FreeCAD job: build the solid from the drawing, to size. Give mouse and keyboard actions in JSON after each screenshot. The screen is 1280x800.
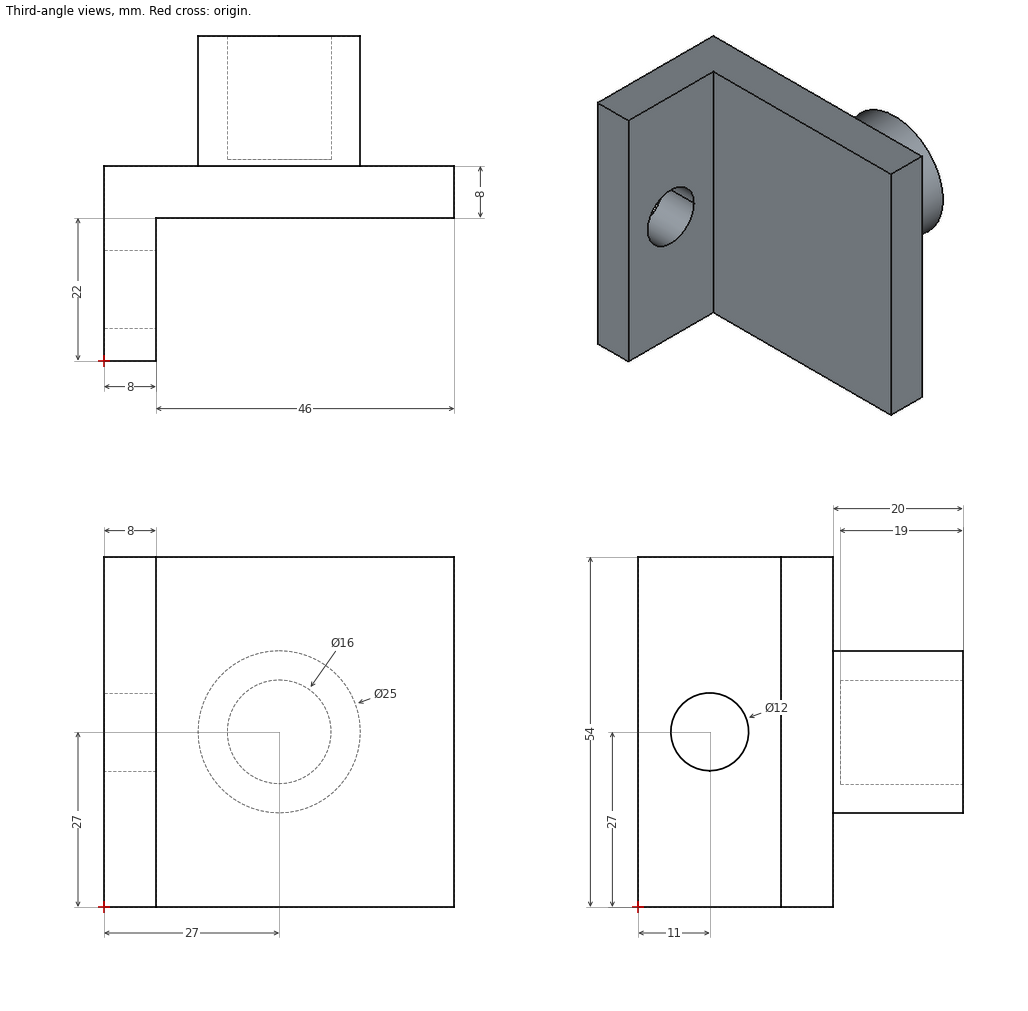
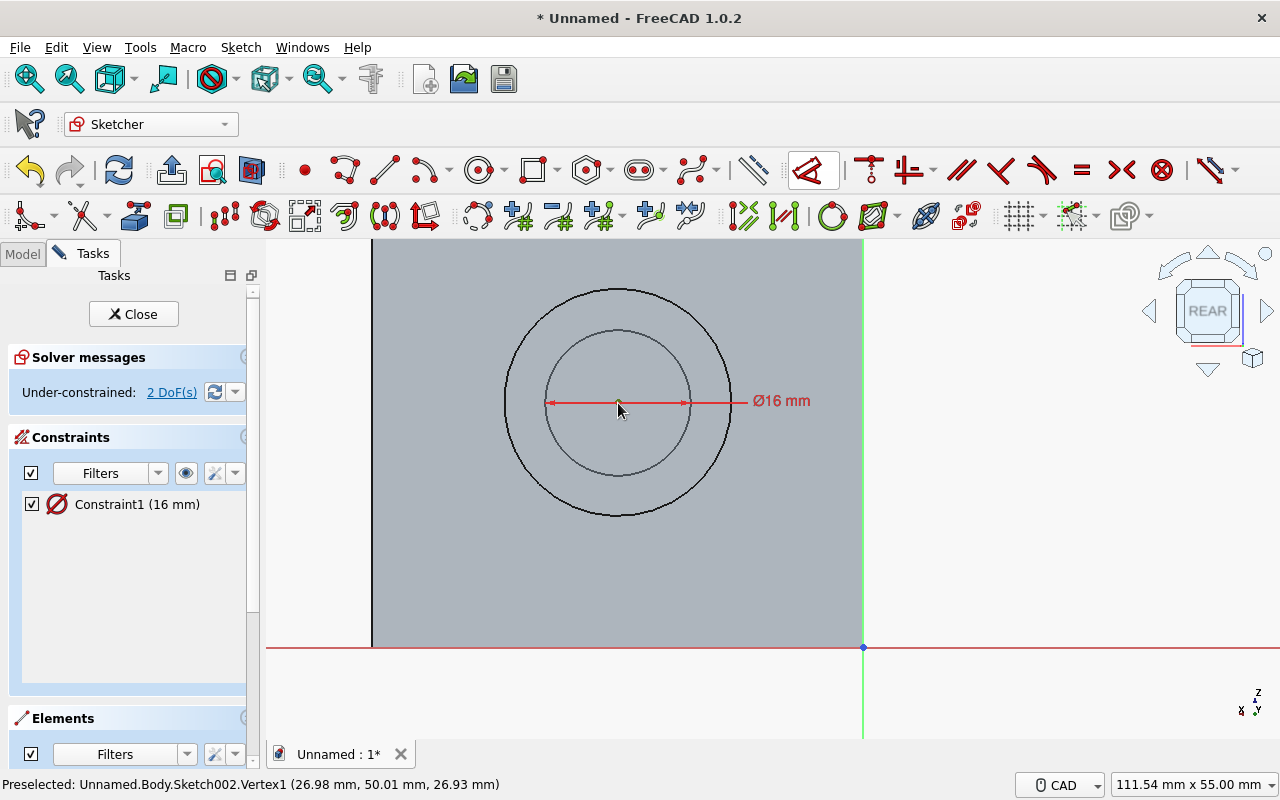
{"action": "key", "text": "l"}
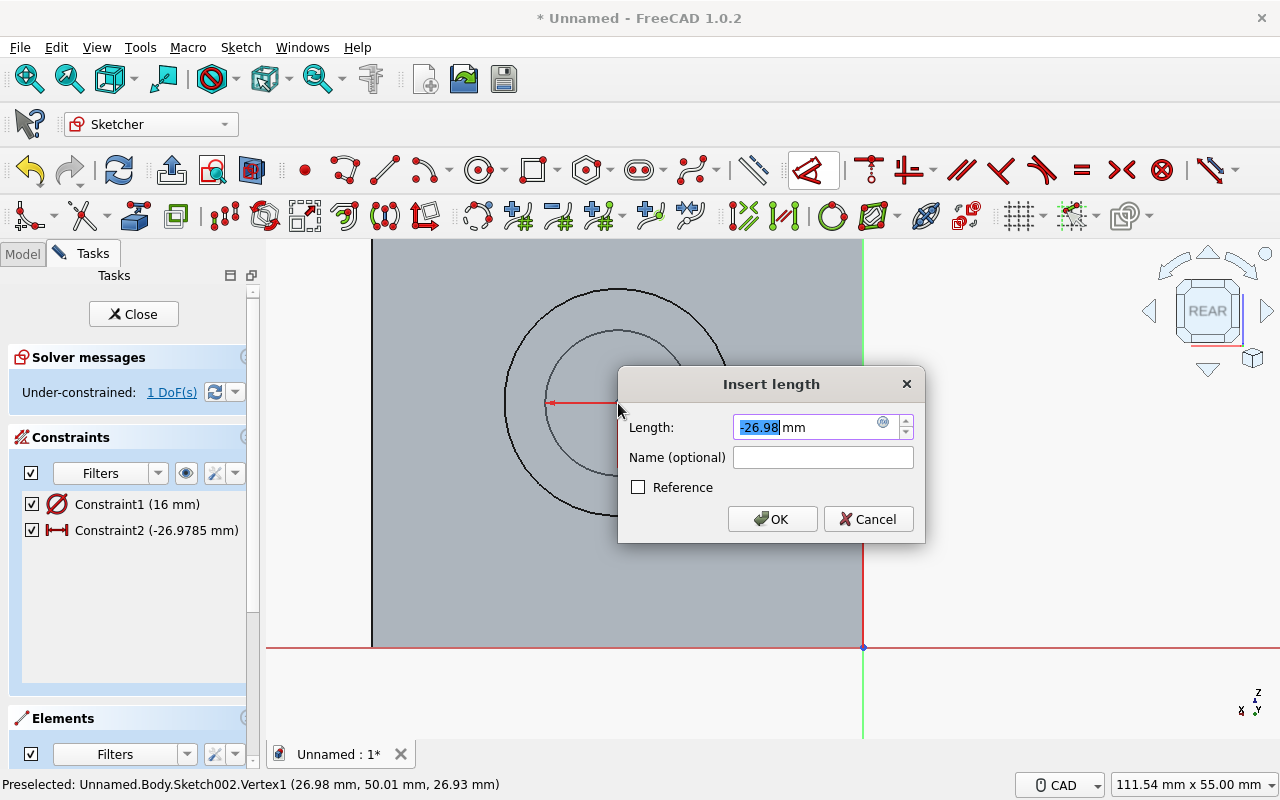
{"action": "type", "text": "-27"}
{"action": "key", "text": "Return"}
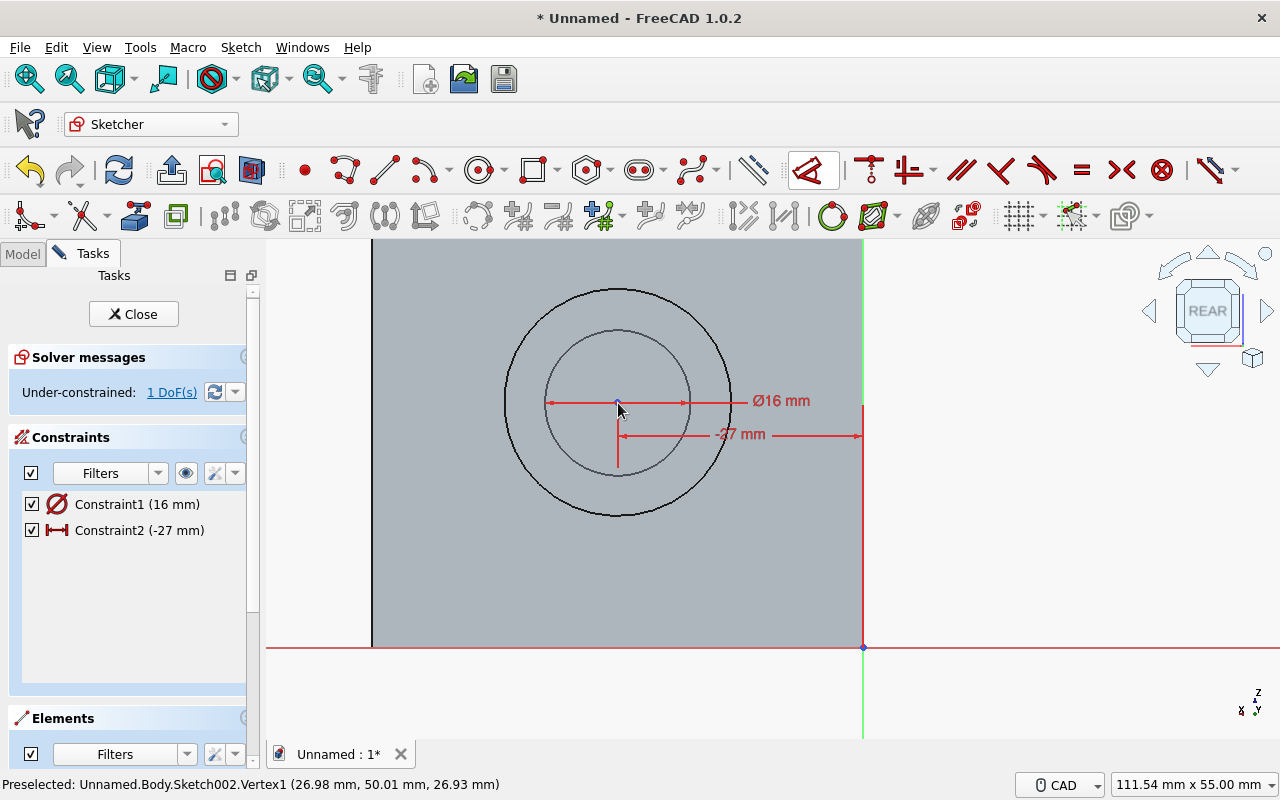
{"action": "left_click", "coordinate": [618, 403]}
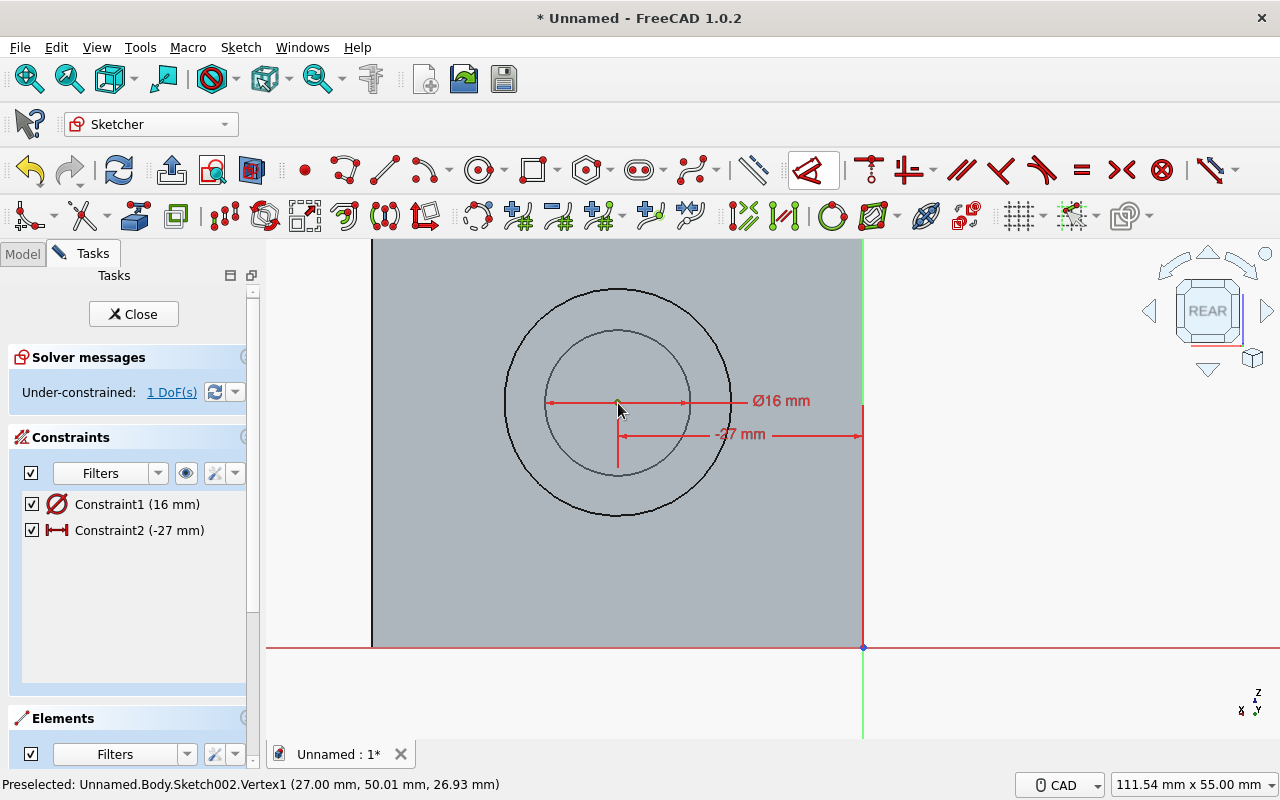
{"action": "key", "text": "i"}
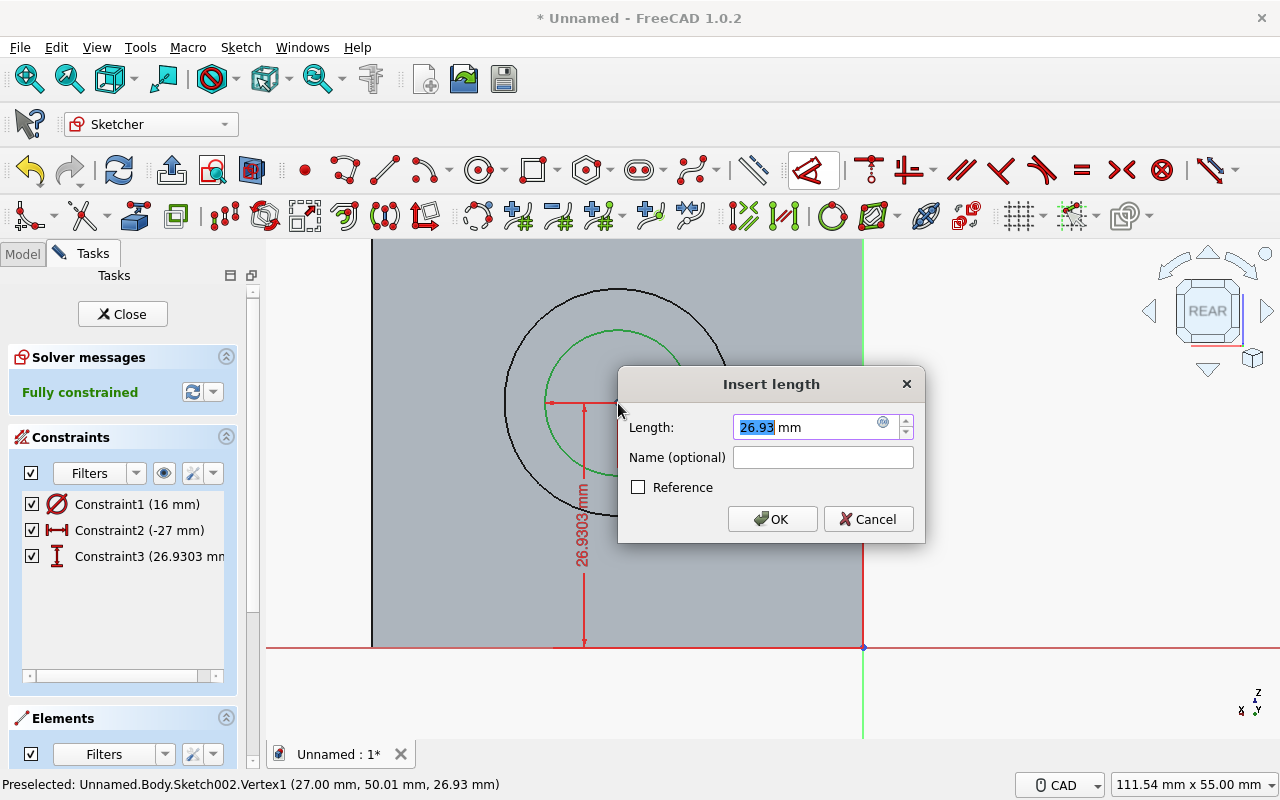
{"action": "type", "text": "27"}
{"action": "key", "text": "Return"}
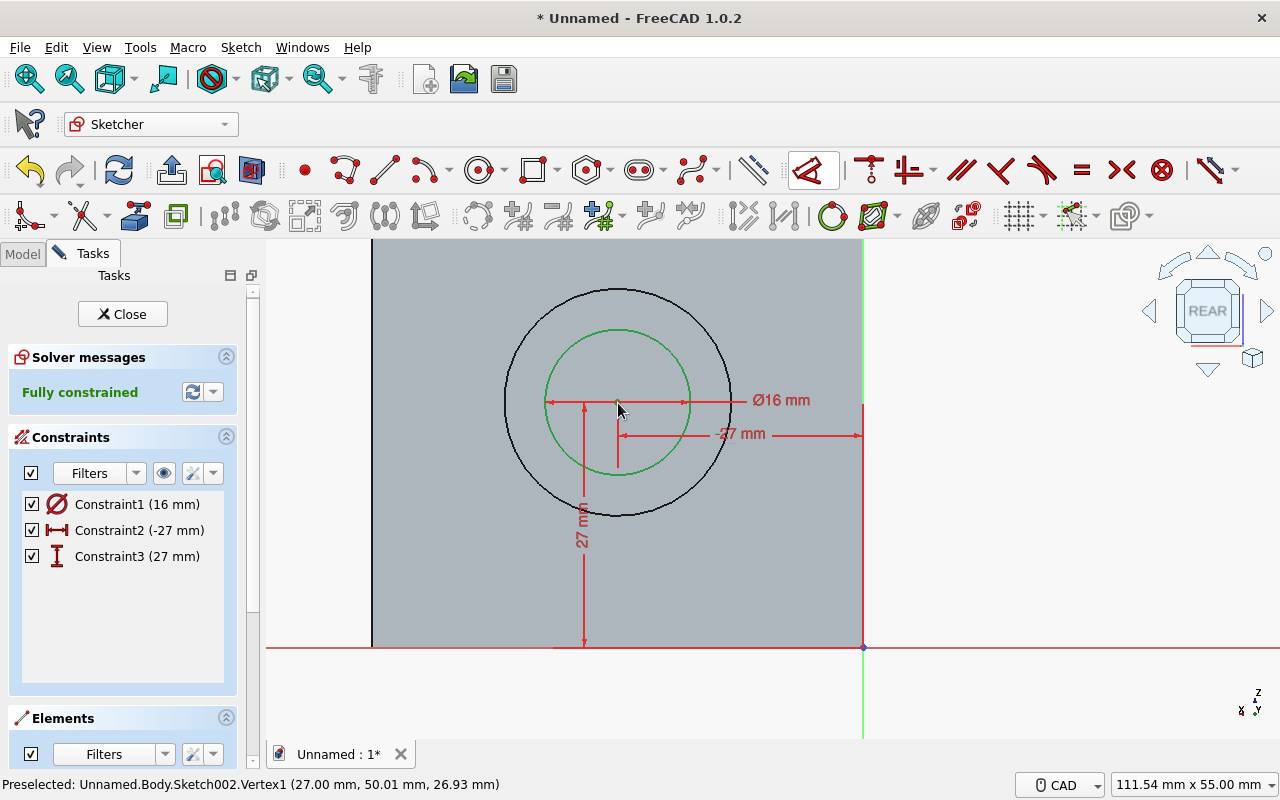
{"action": "left_click", "coordinate": [123, 314]}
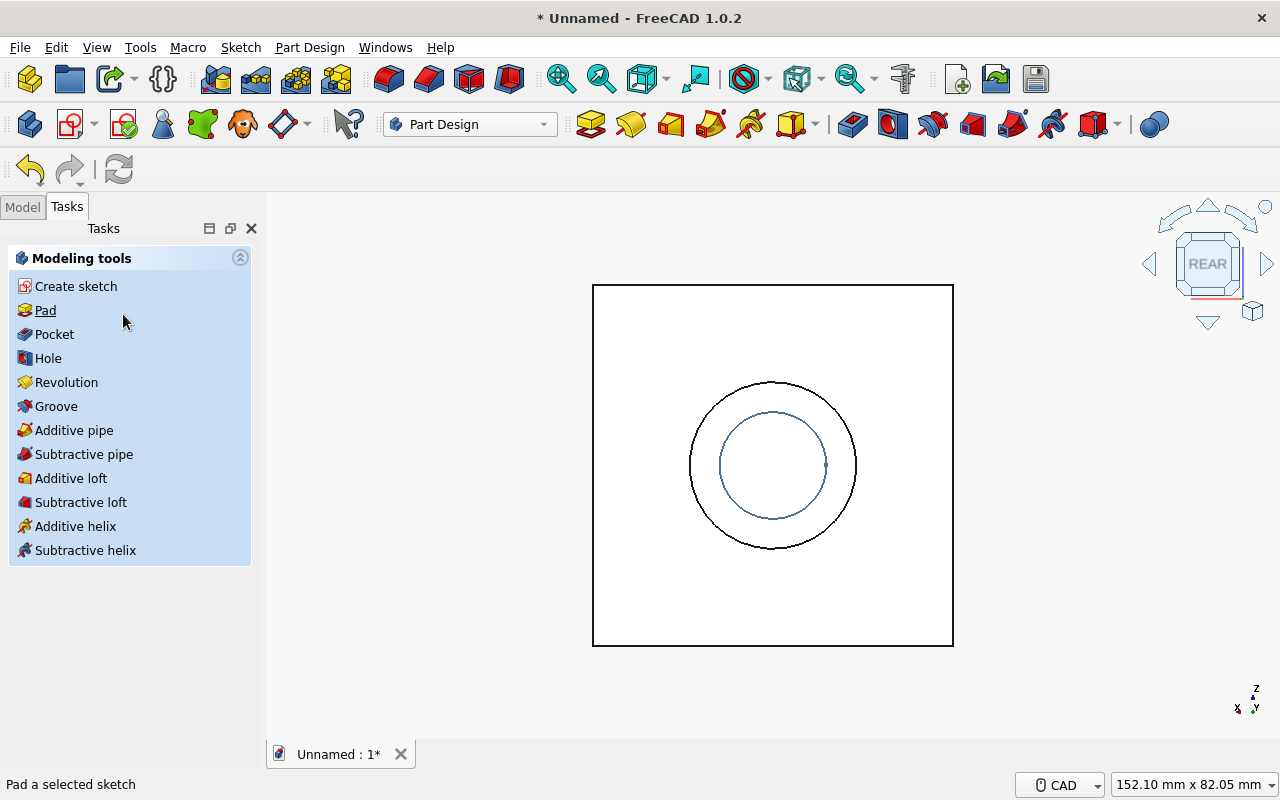
{"action": "left_click", "coordinate": [854, 124]}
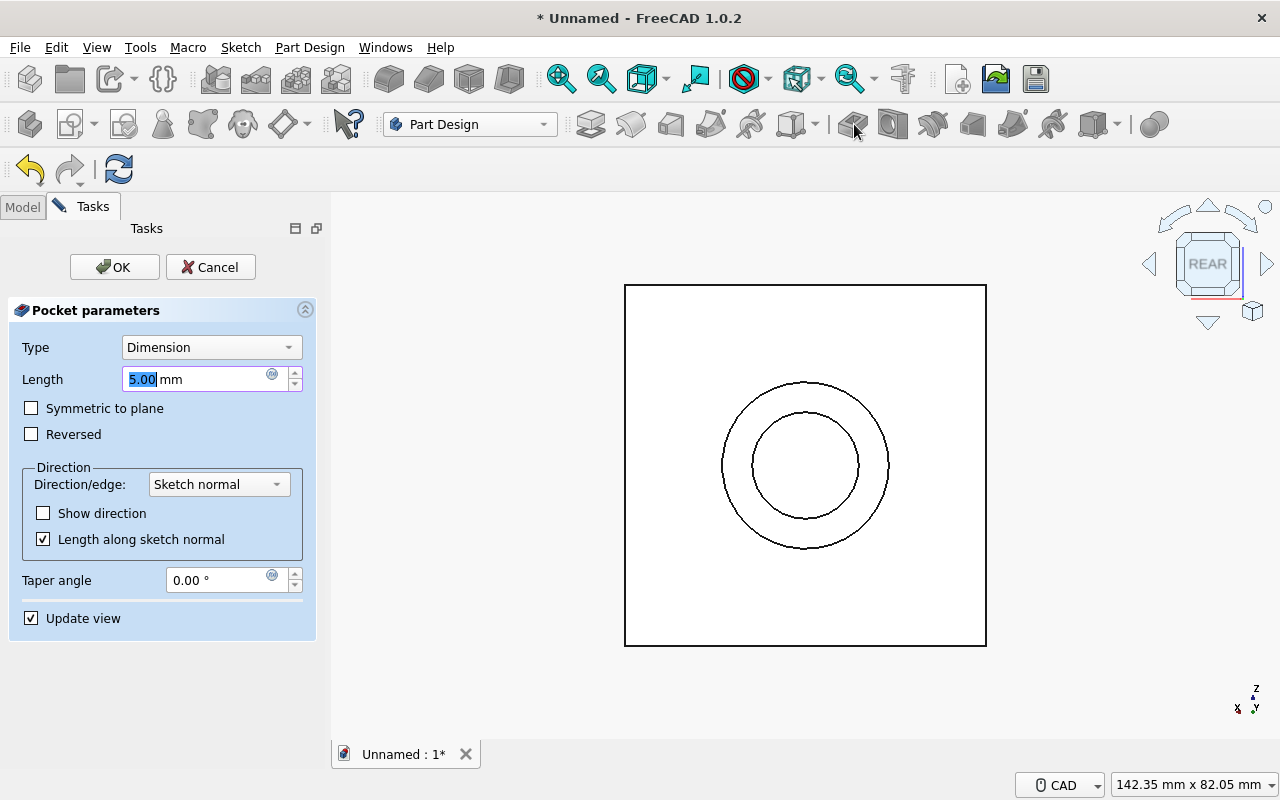
{"action": "type", "text": "19"}
{"action": "key", "text": "Tab"}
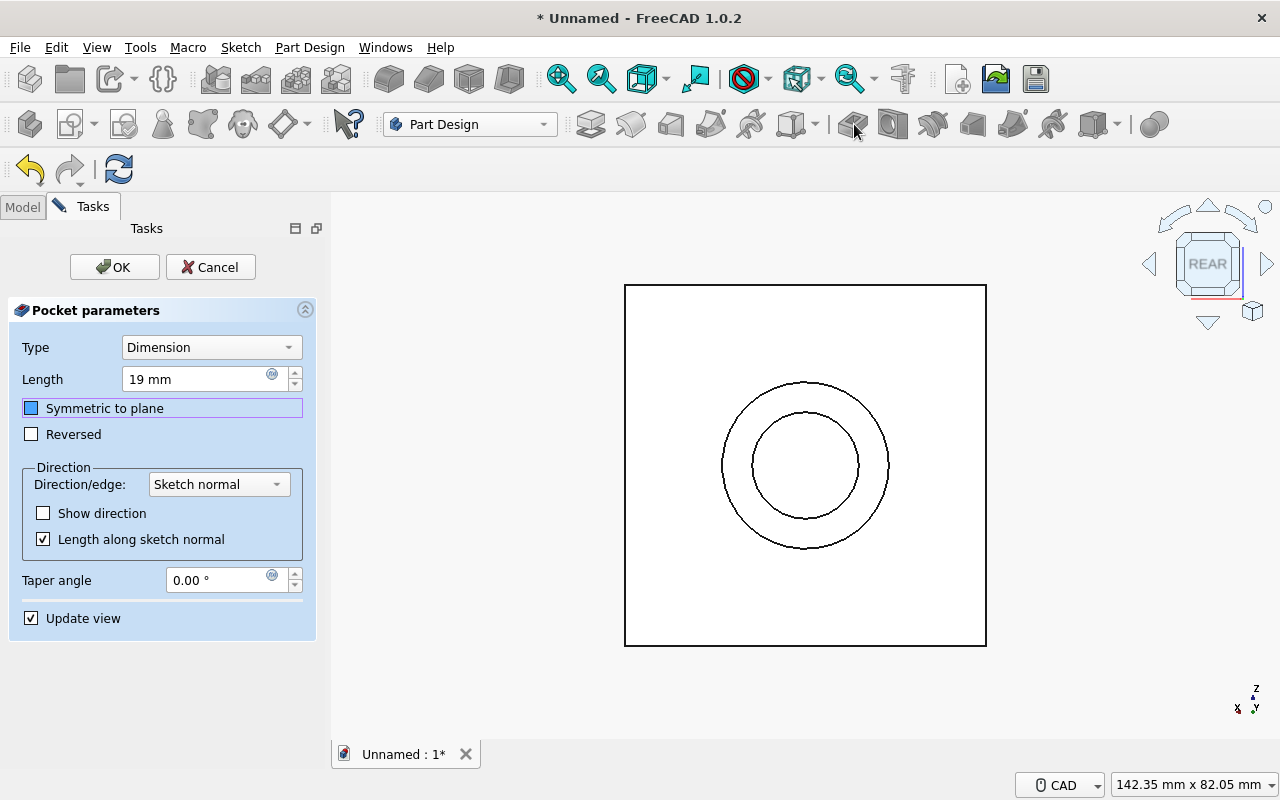
{"action": "left_click", "coordinate": [115, 267]}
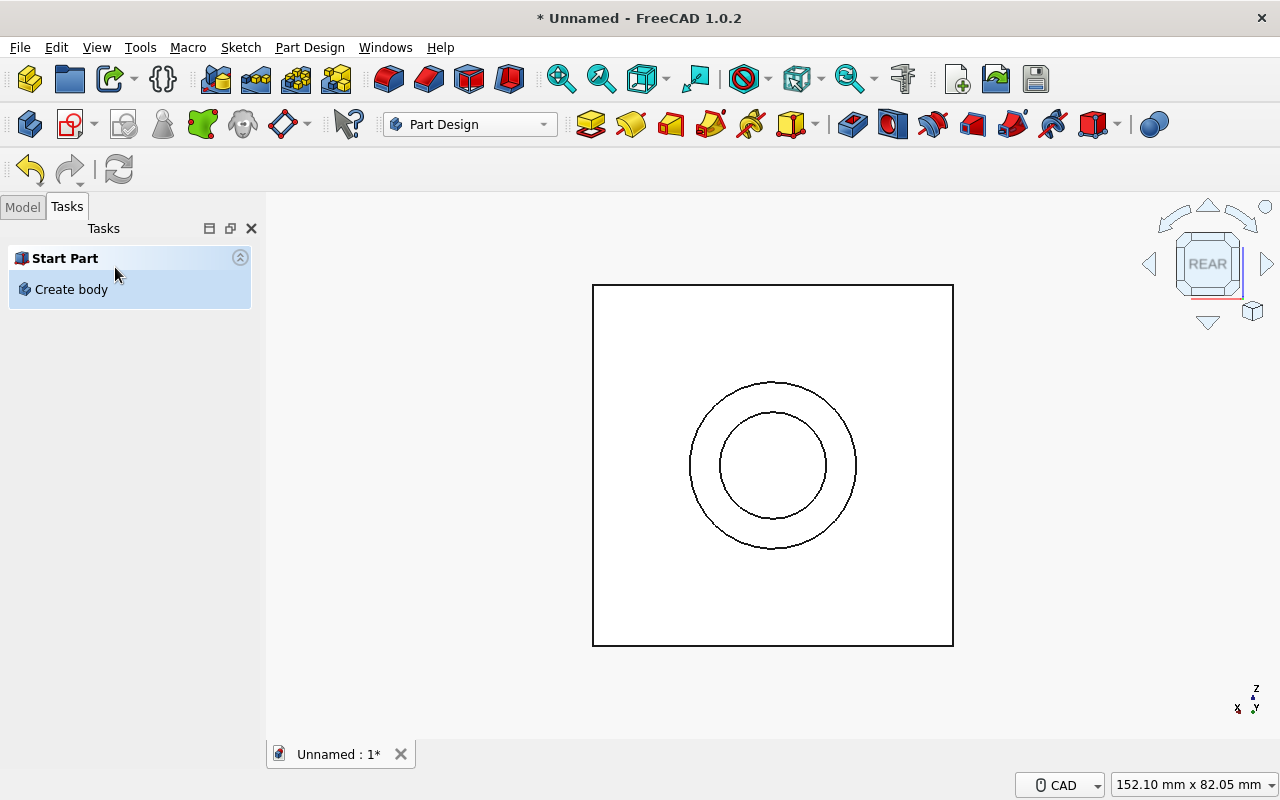
{"action": "key", "text": "0"}